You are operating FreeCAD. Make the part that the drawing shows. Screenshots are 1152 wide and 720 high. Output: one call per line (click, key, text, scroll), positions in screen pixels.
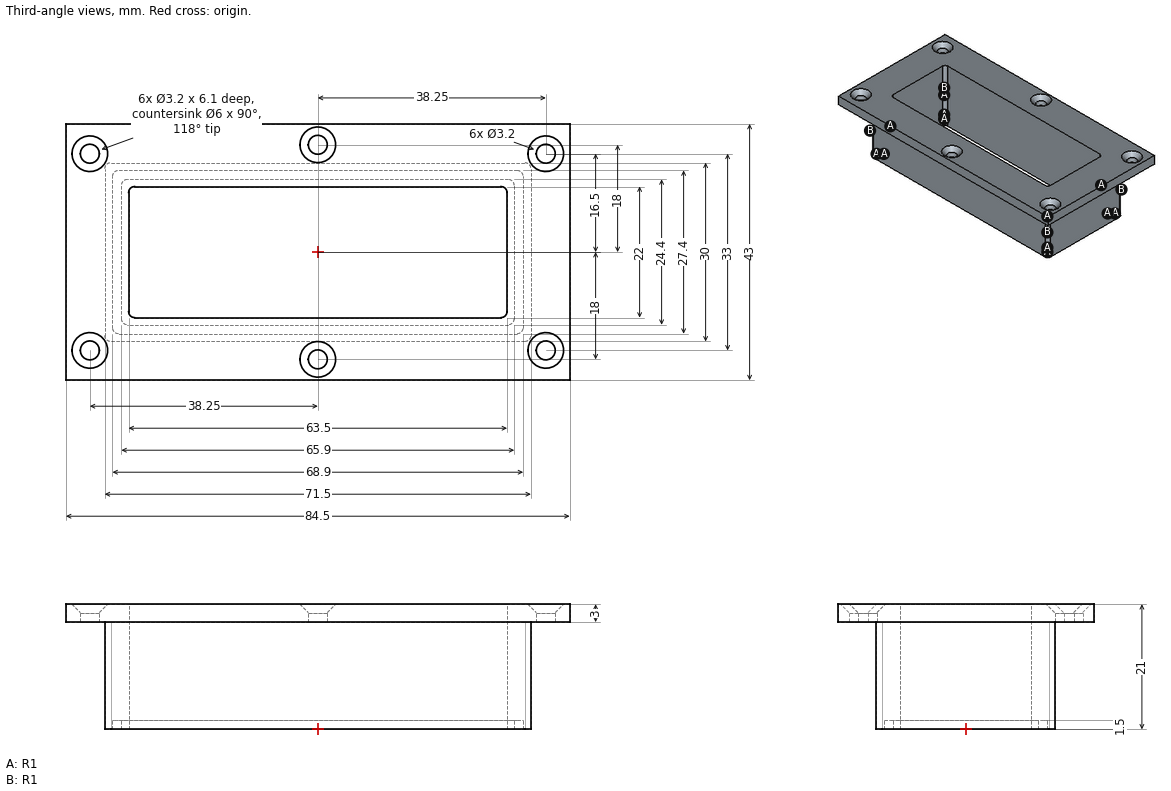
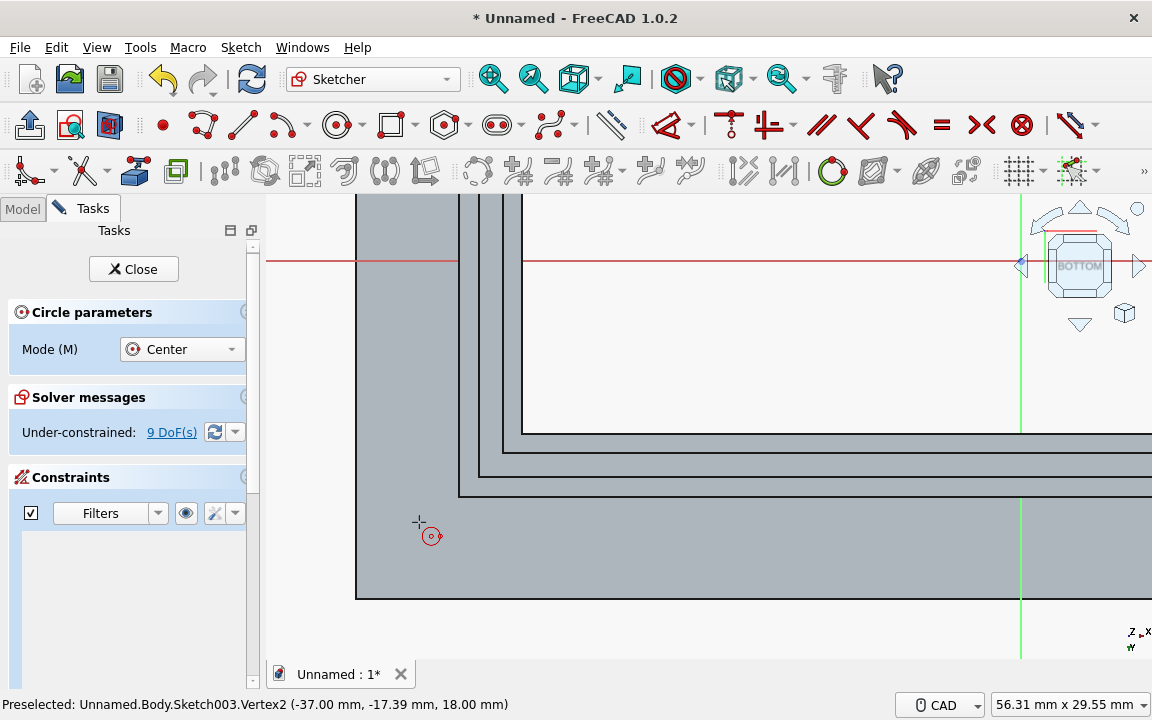
click(419, 521)
click(437, 503)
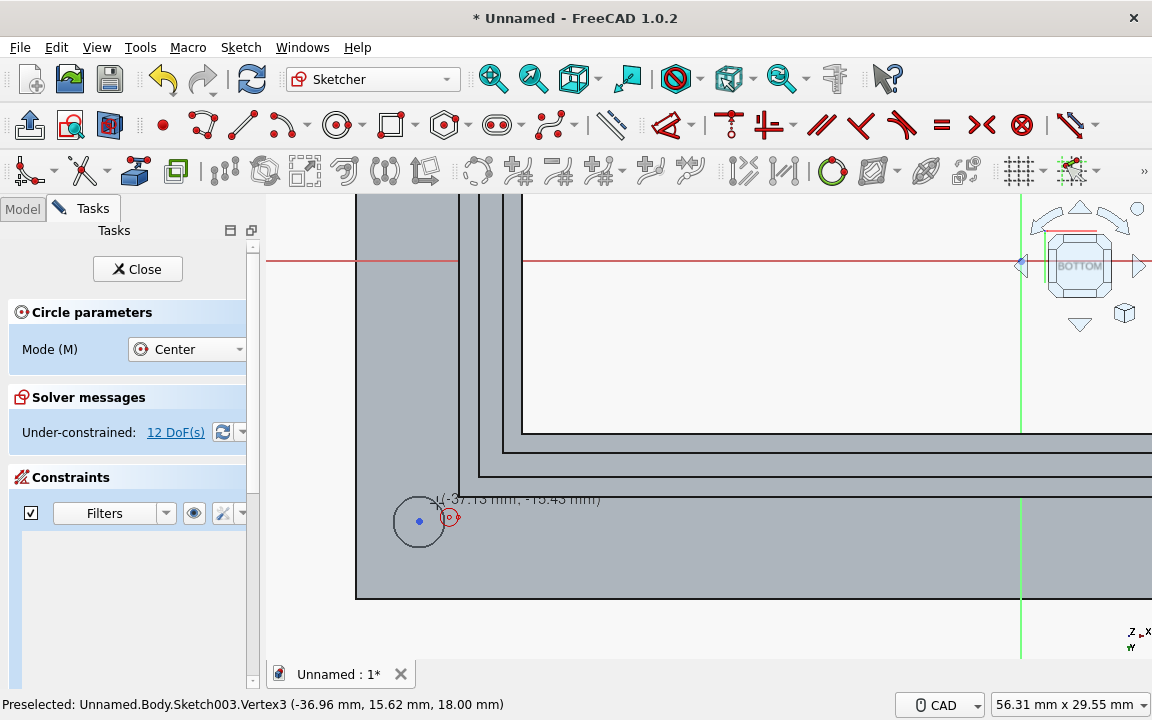
scroll(419, 523, down, 5)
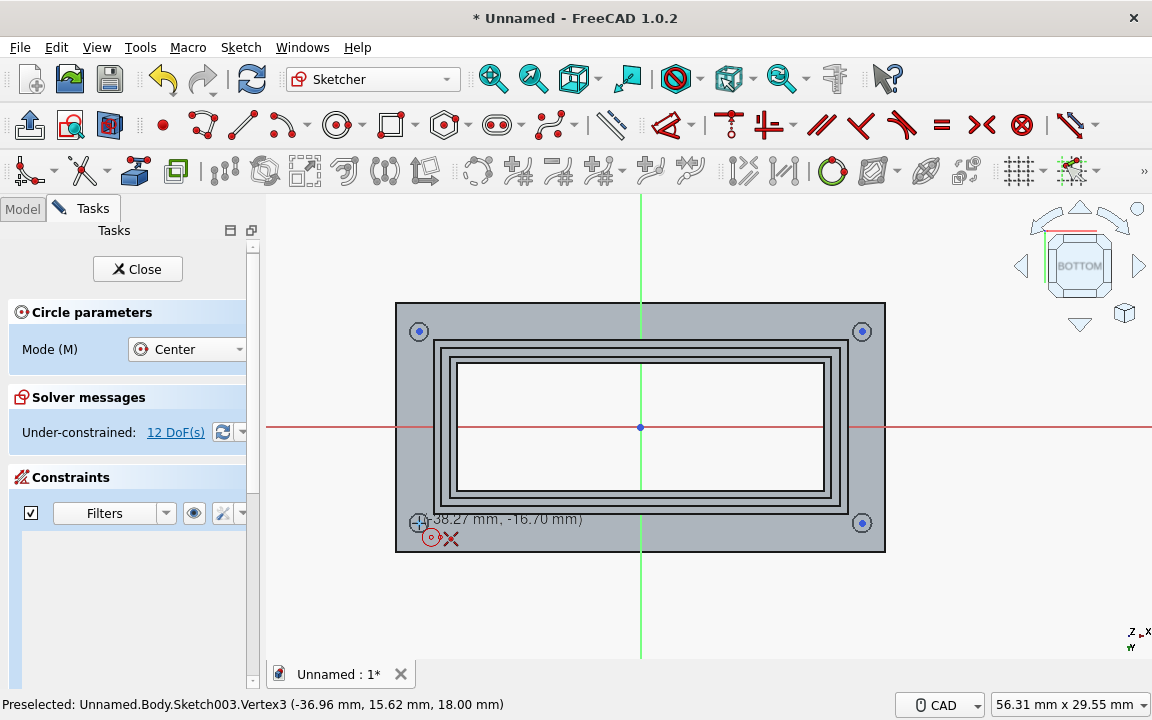
scroll(641, 323, up, 5)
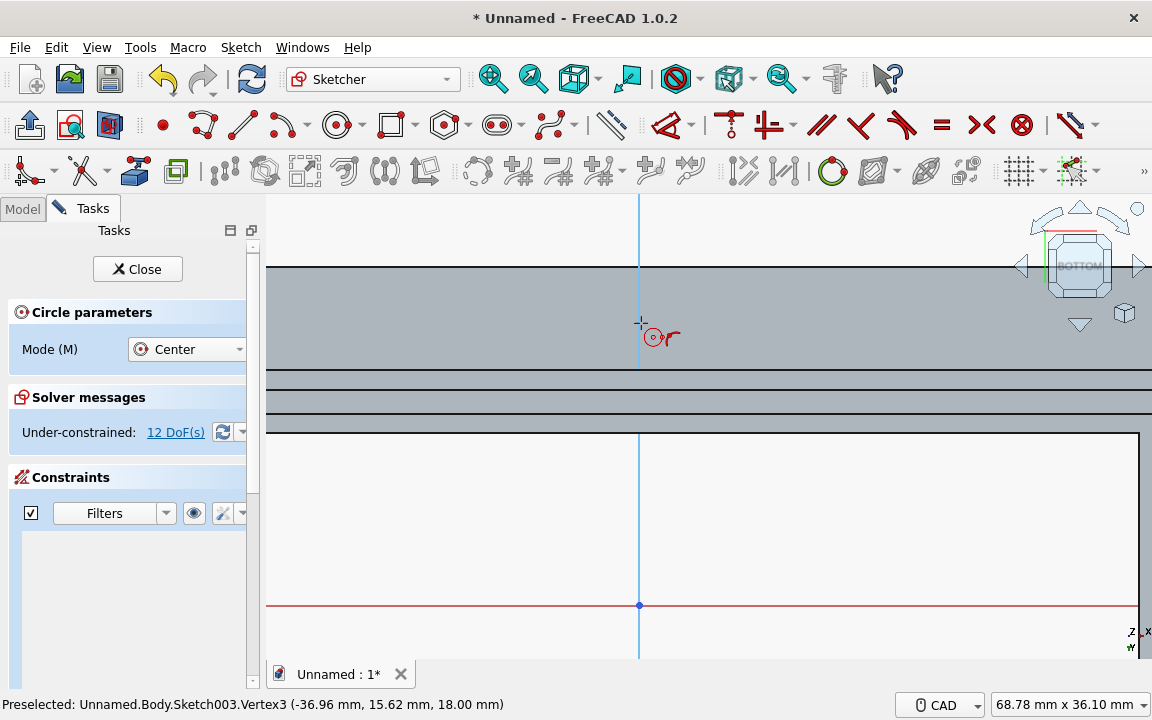
click(639, 322)
click(657, 305)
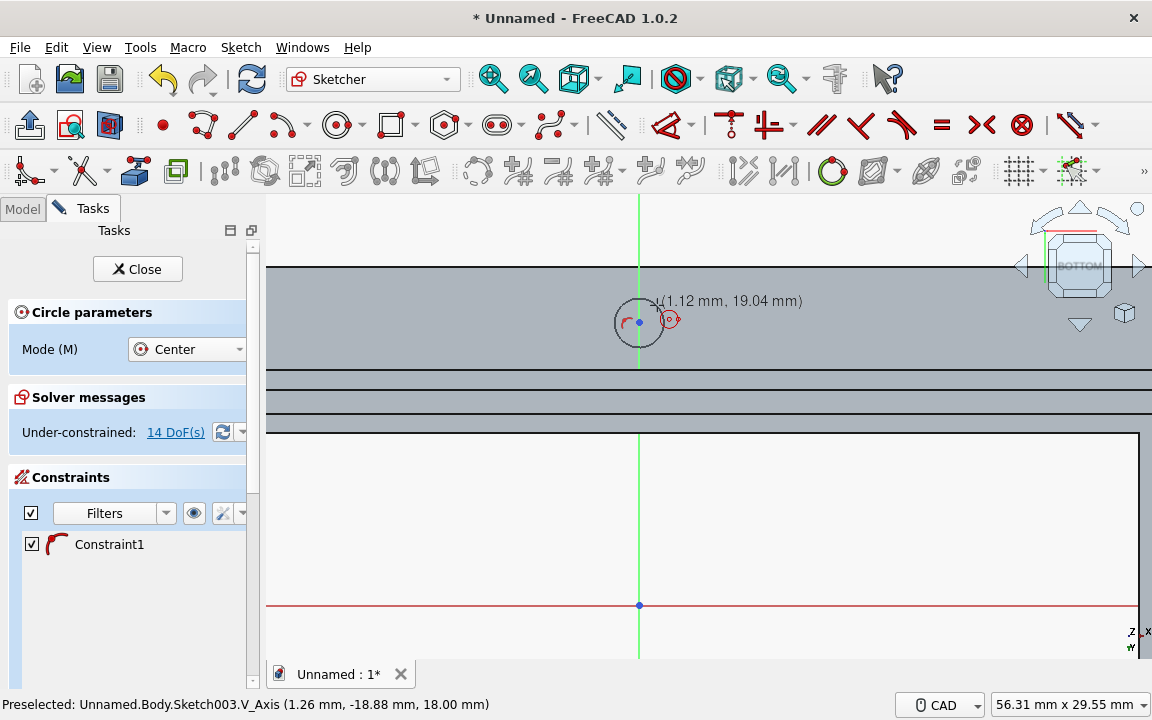
scroll(641, 322, down, 5)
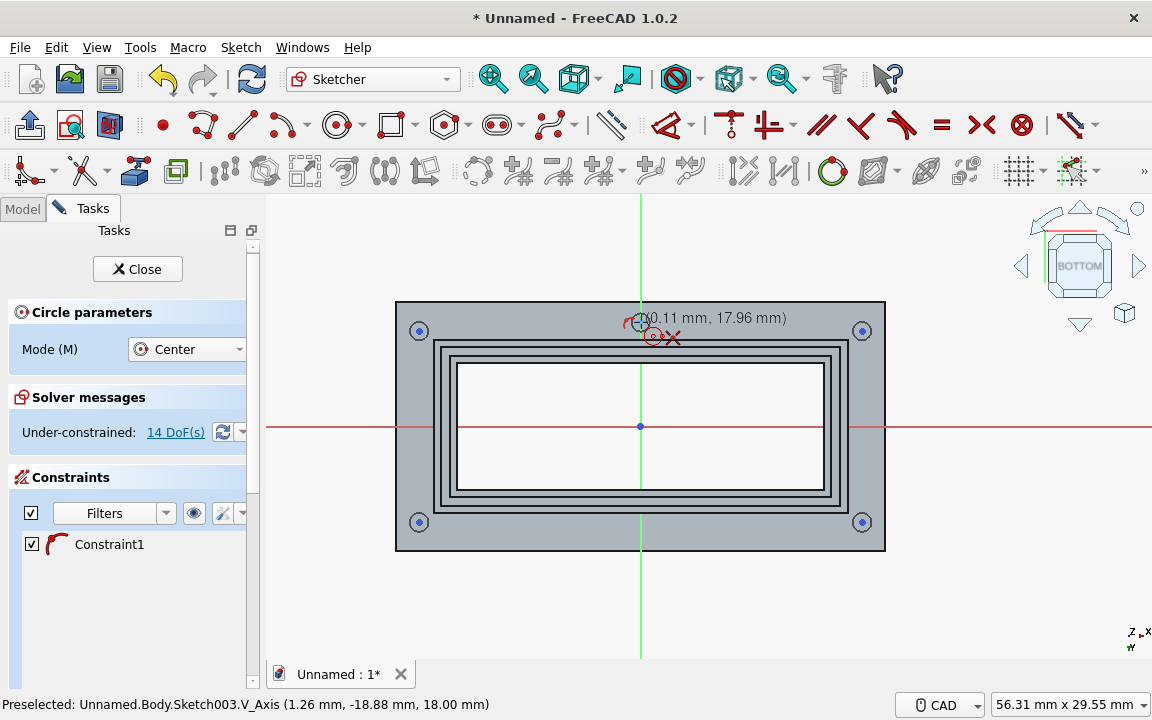
scroll(641, 531, up, 5)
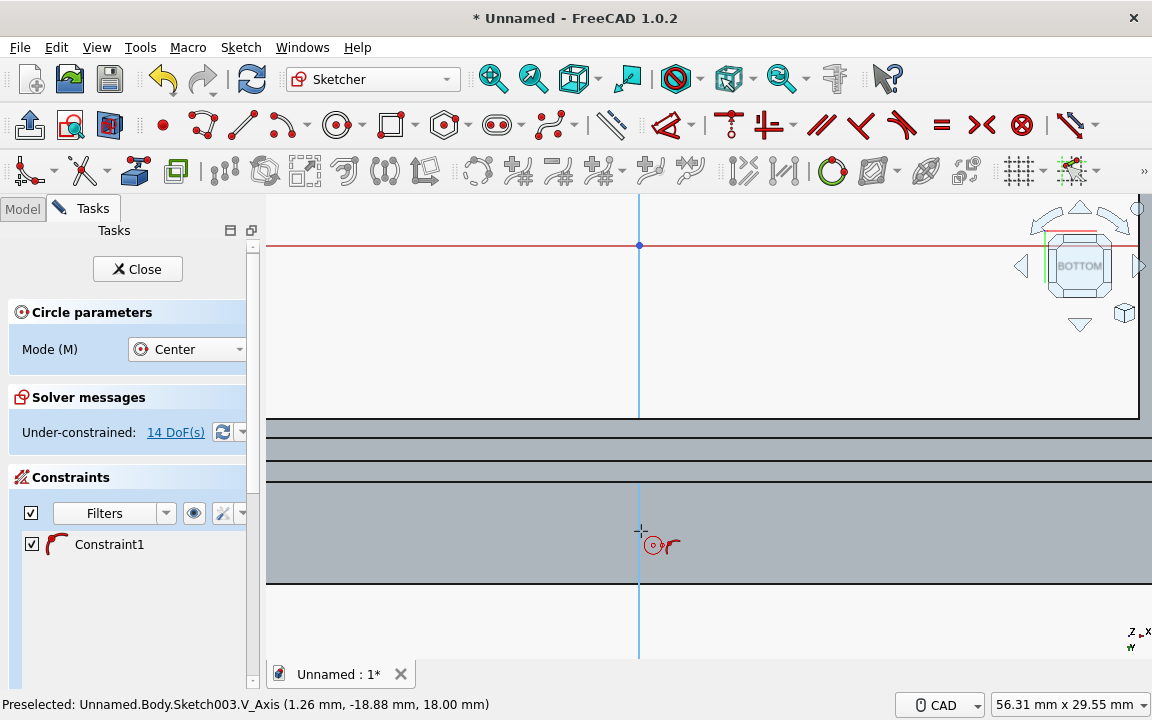
click(639, 529)
click(657, 511)
key(Escape)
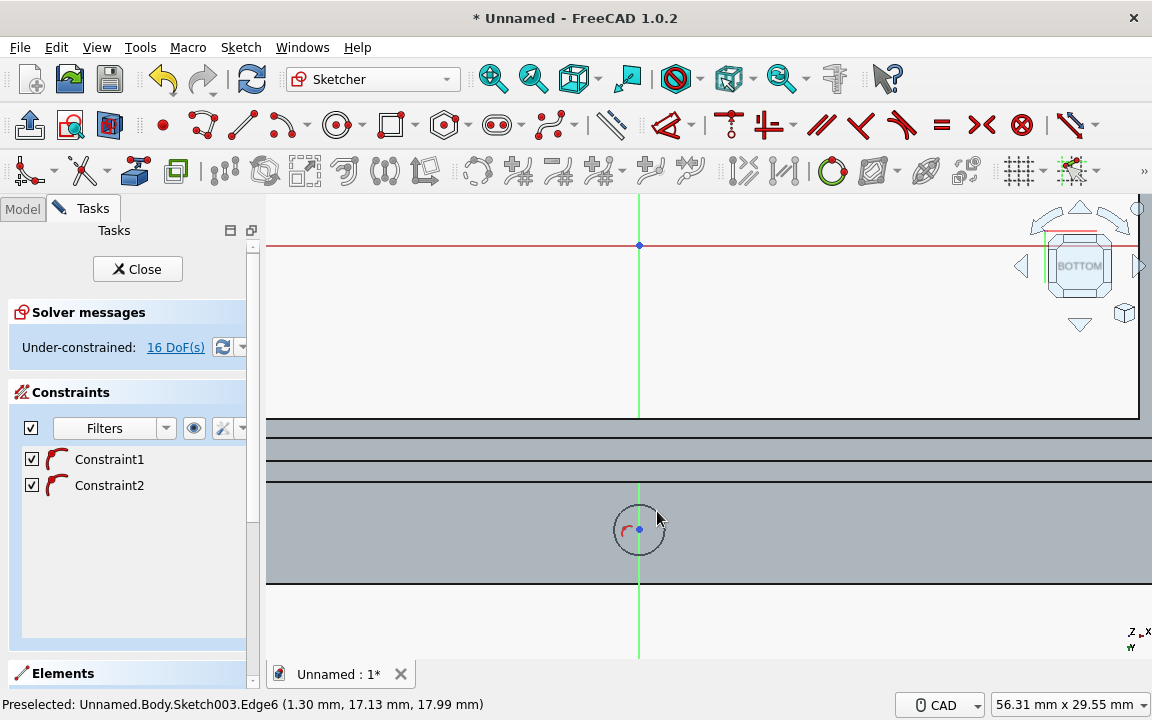
scroll(641, 532, down, 5)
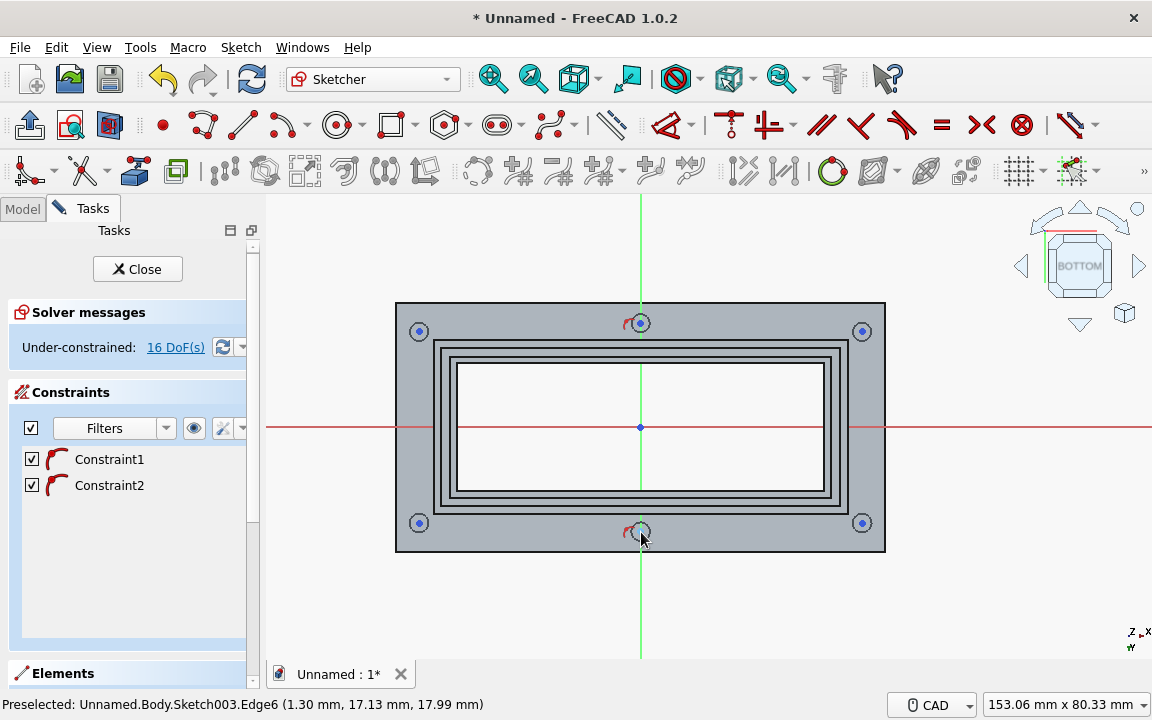
scroll(869, 516, up, 2)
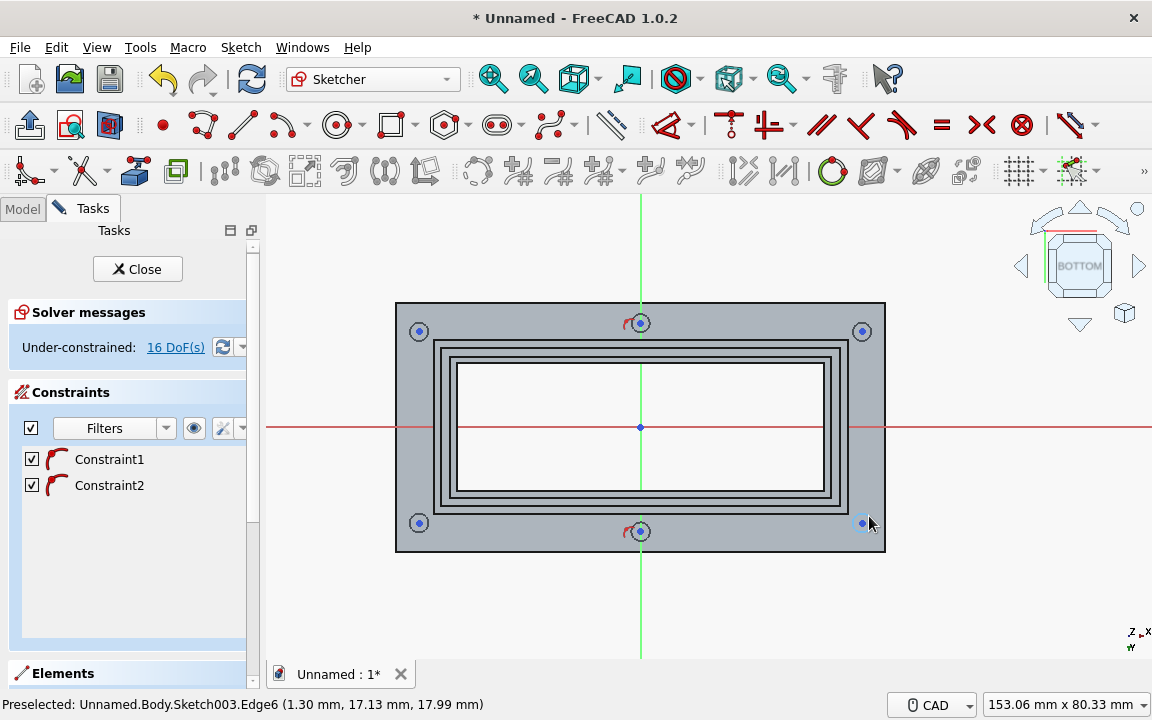
click(868, 516)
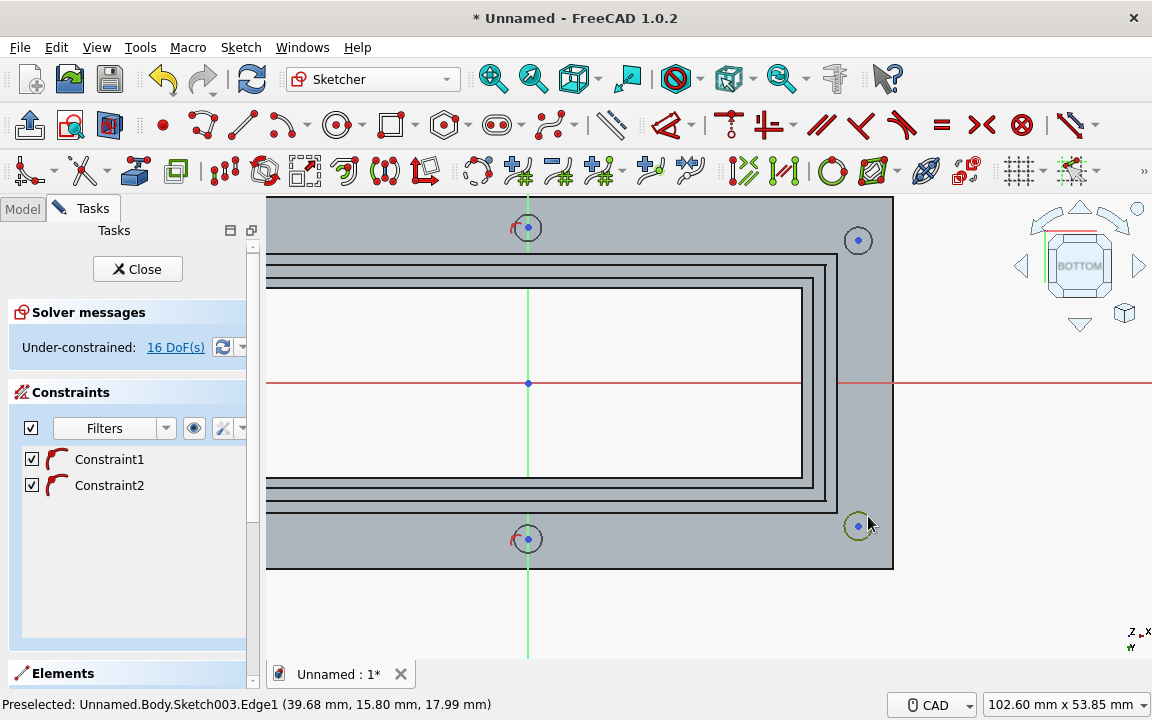
click(868, 231)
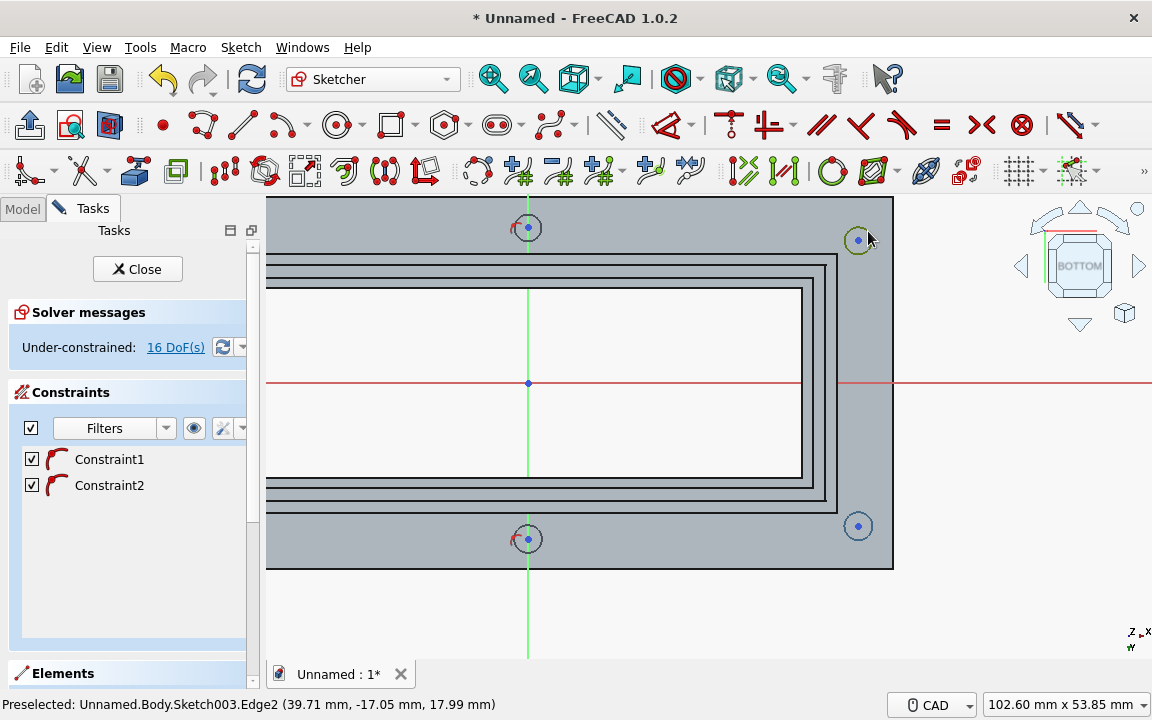
scroll(869, 515, down, 2)